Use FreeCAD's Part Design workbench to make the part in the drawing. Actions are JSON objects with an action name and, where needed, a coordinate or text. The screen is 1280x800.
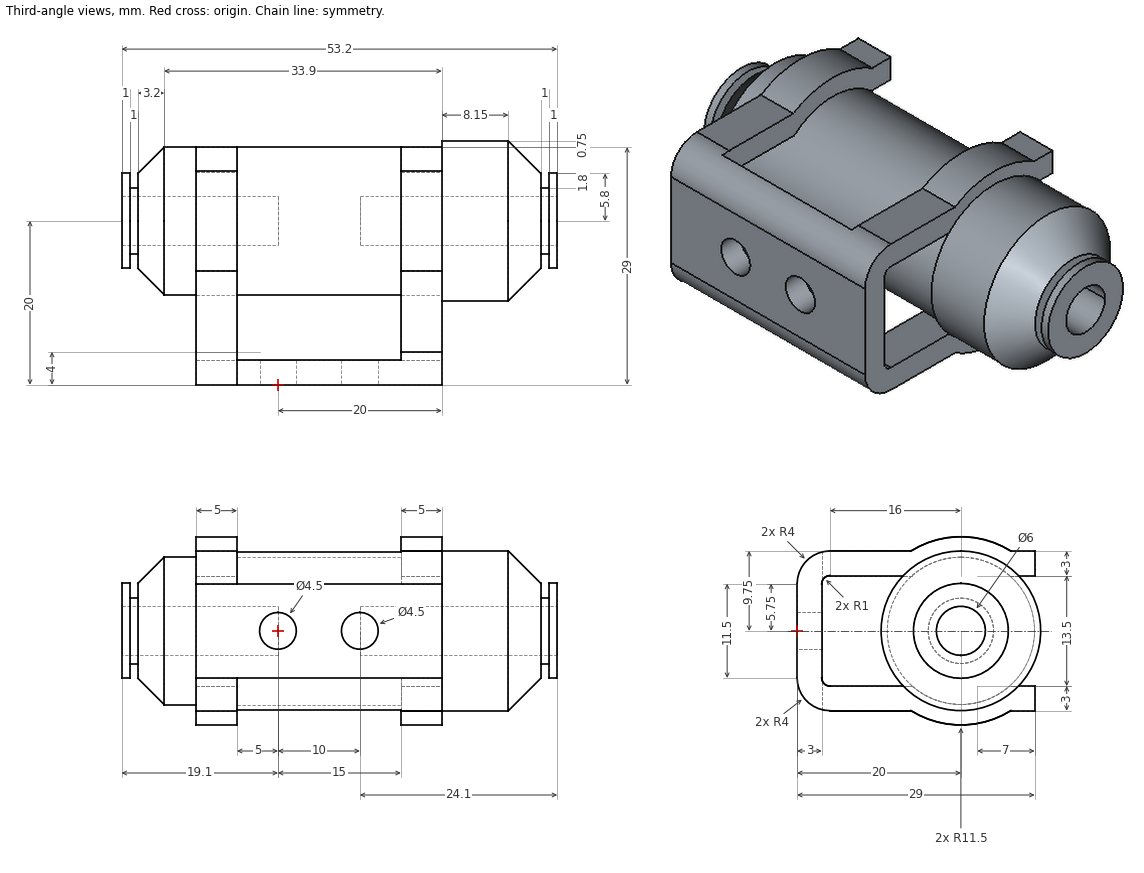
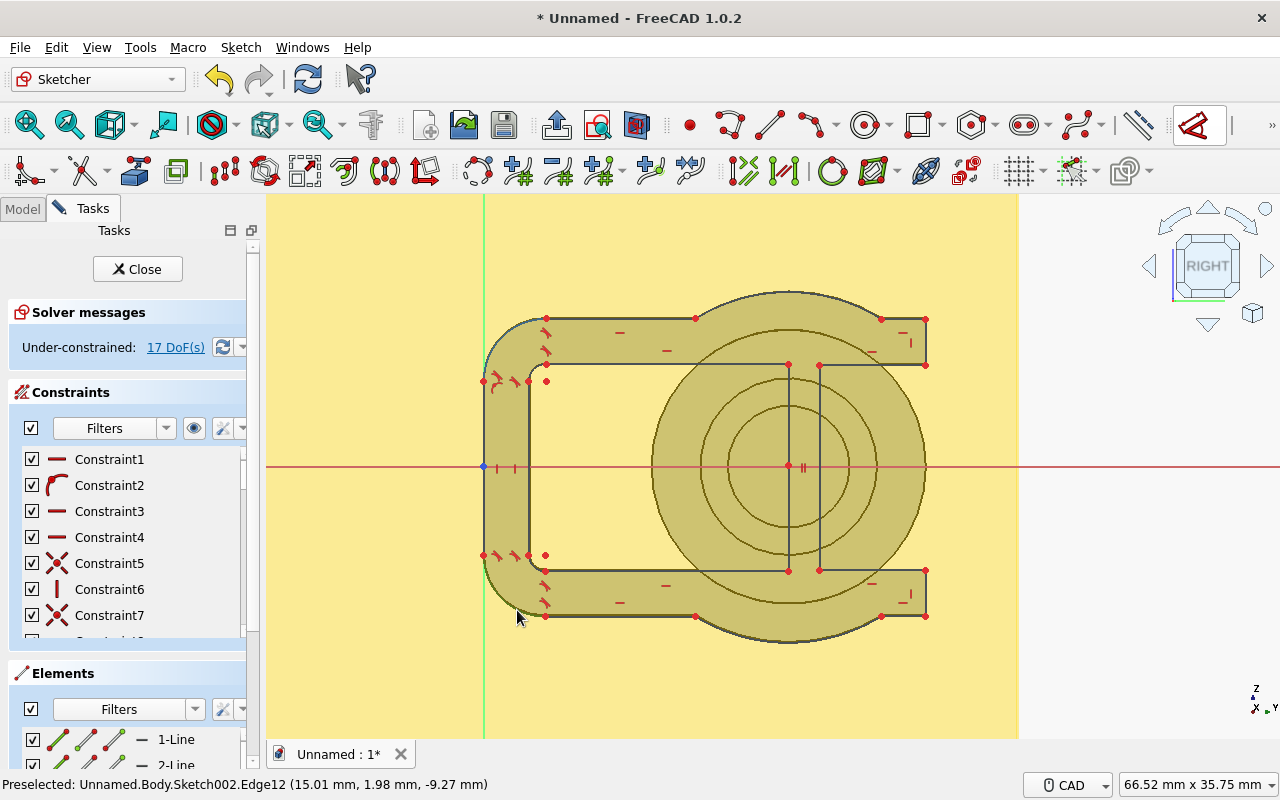
{"action": "key", "text": "e"}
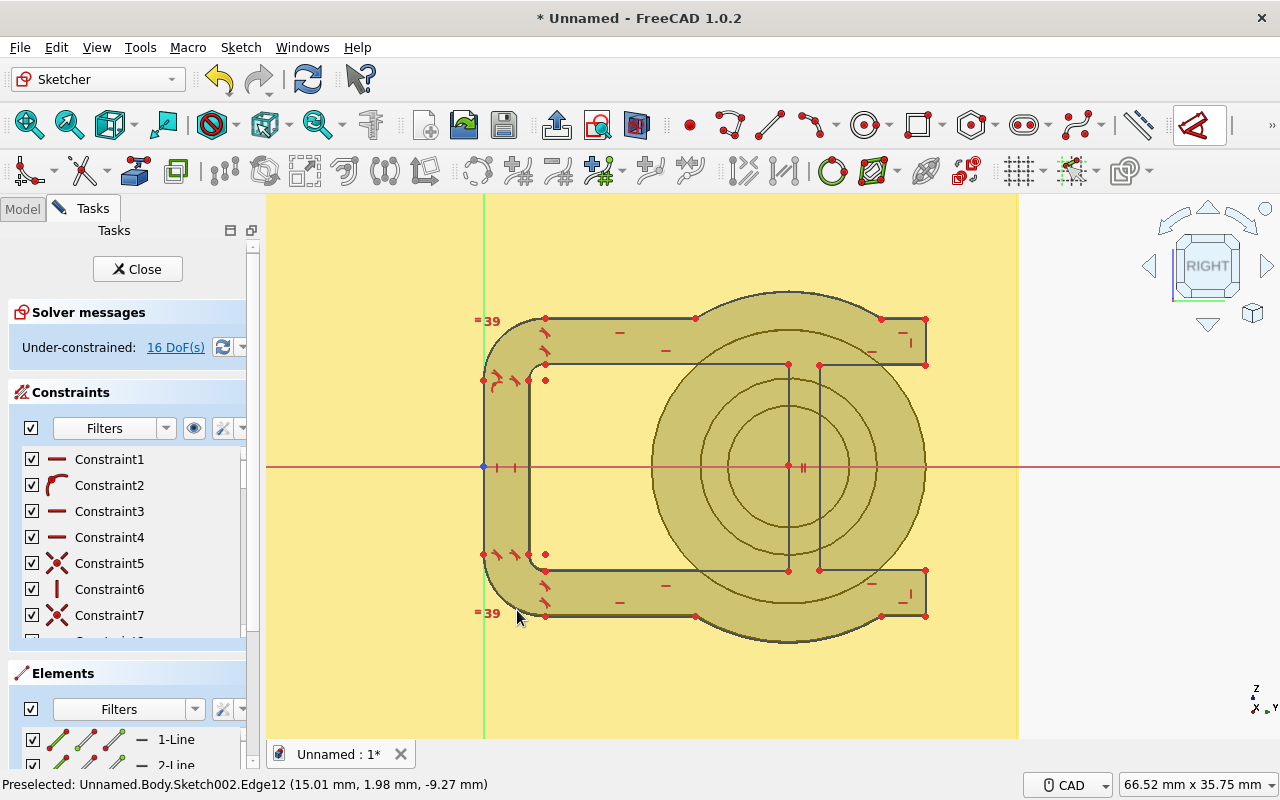
{"action": "left_click", "coordinate": [750, 639]}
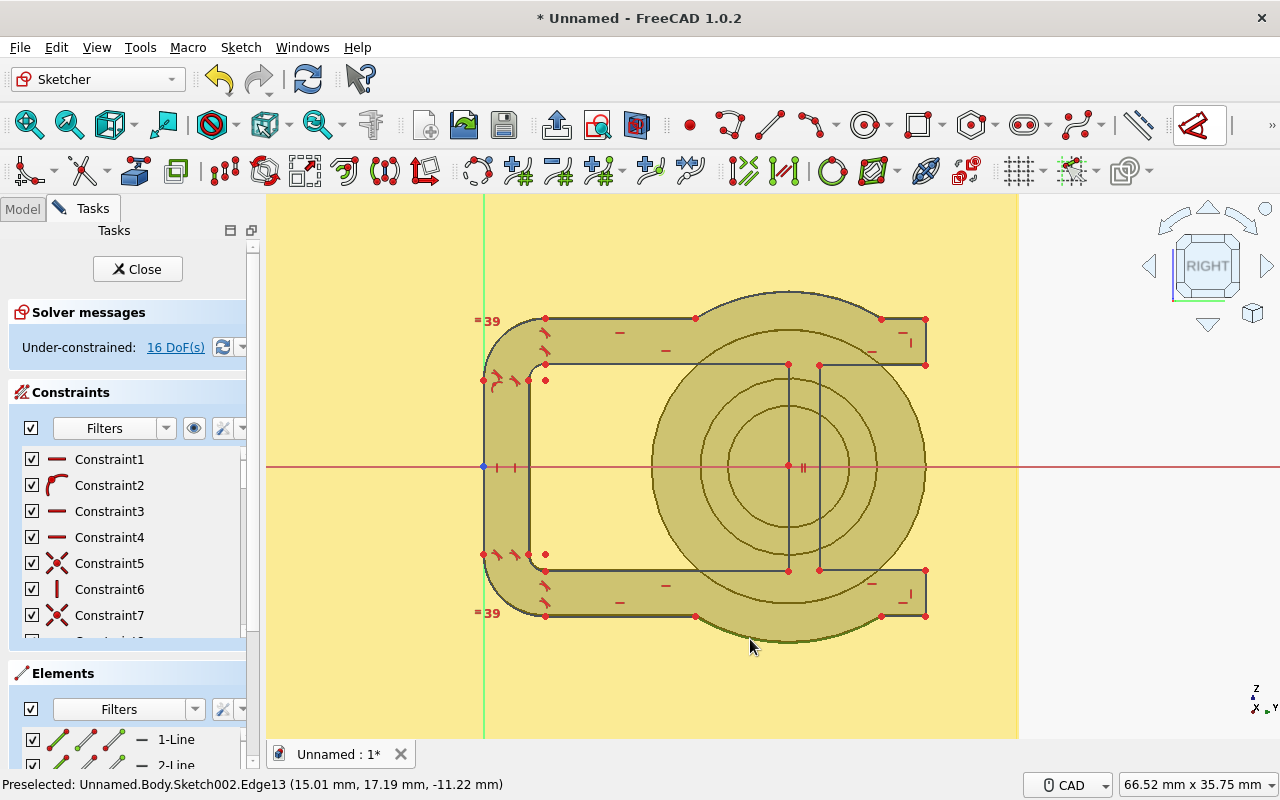
{"action": "left_click", "coordinate": [827, 297]}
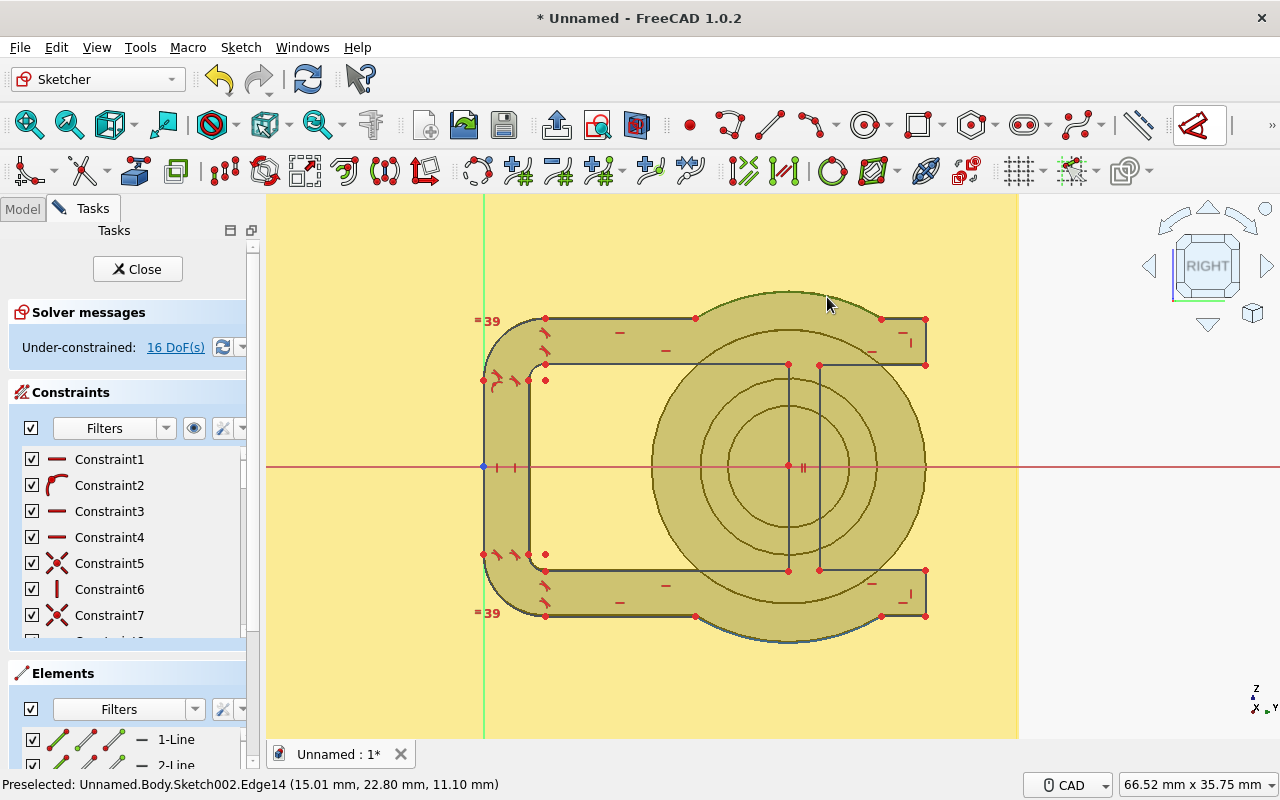
{"action": "key", "text": "e"}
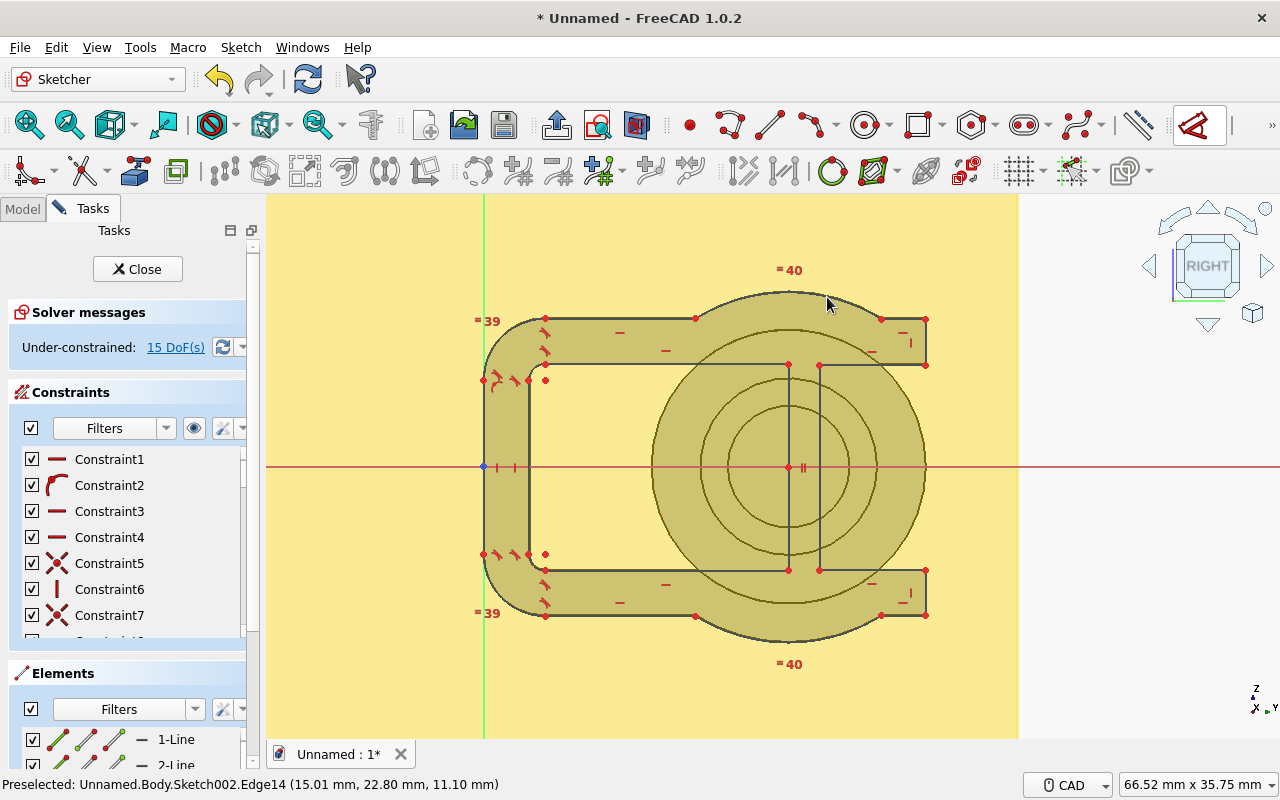
{"action": "left_click", "coordinate": [788, 467]}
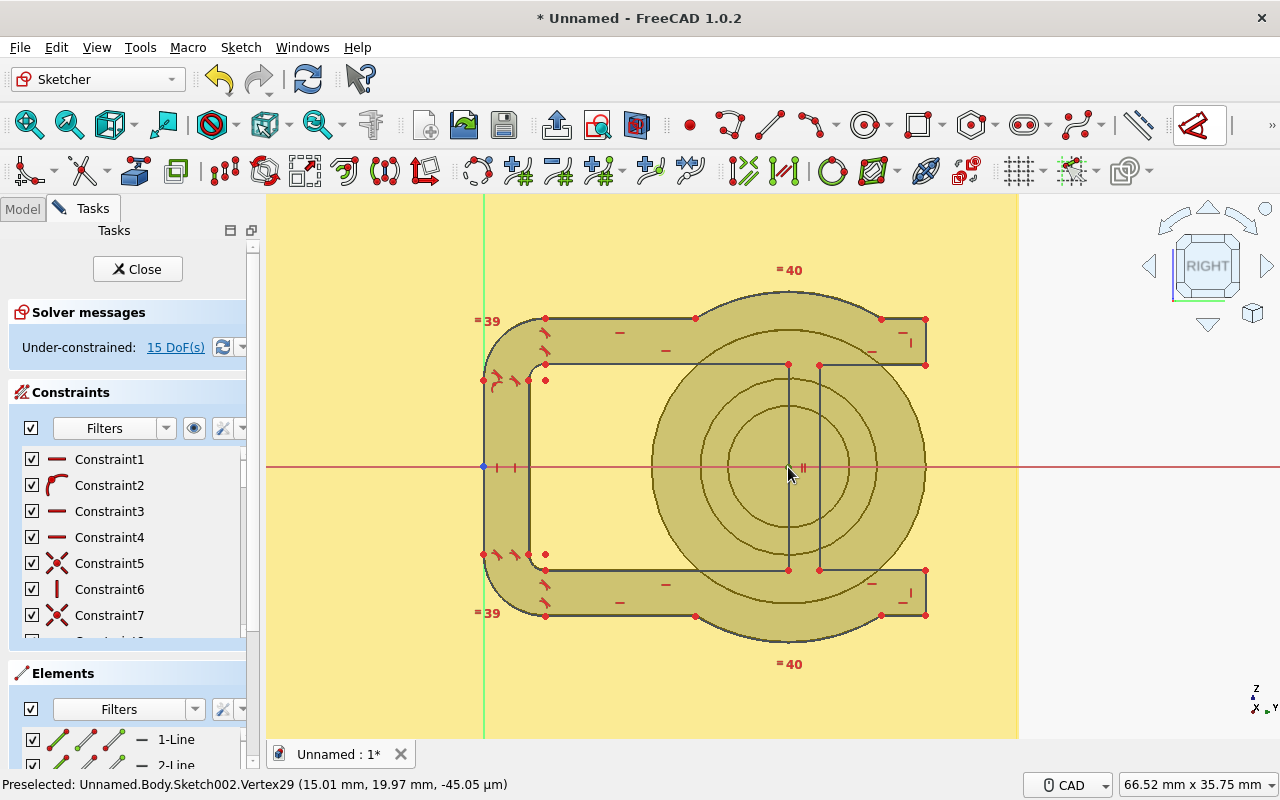
{"action": "left_click", "coordinate": [353, 467]}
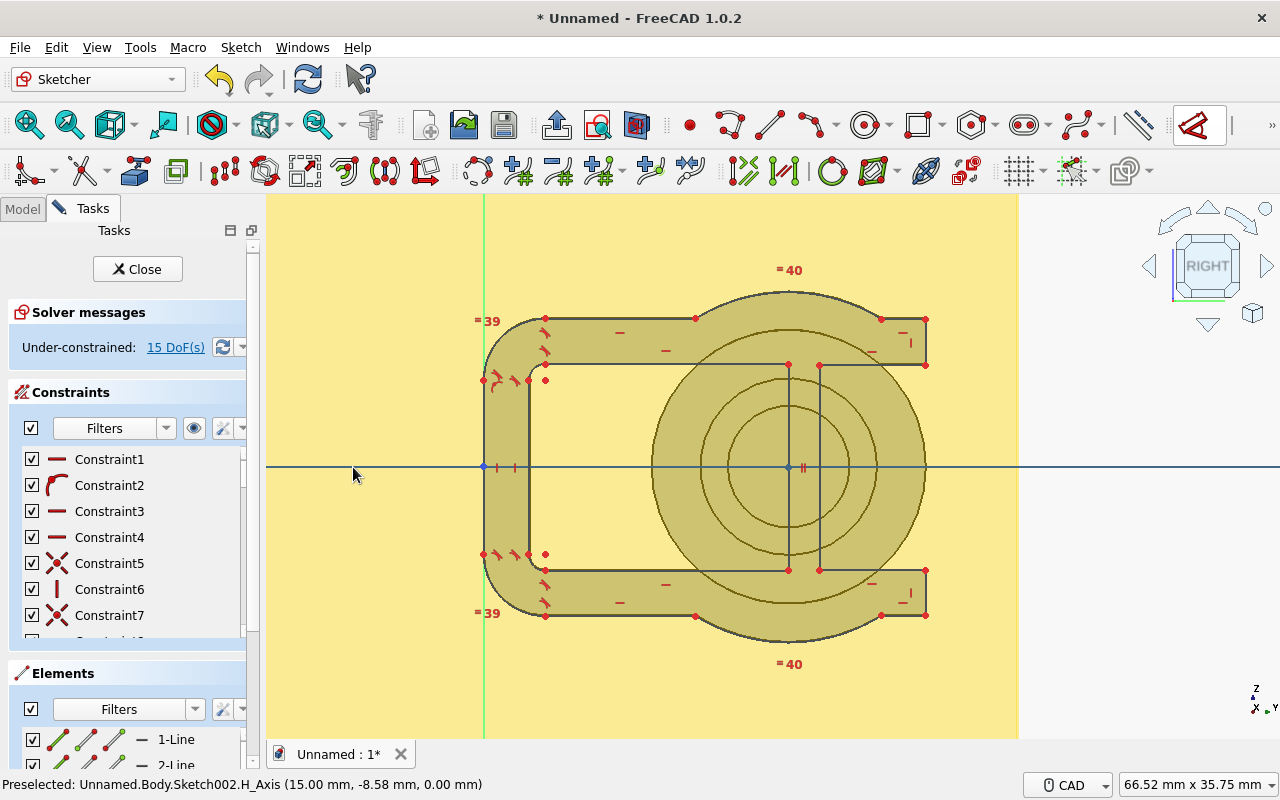
{"action": "key", "text": "c"}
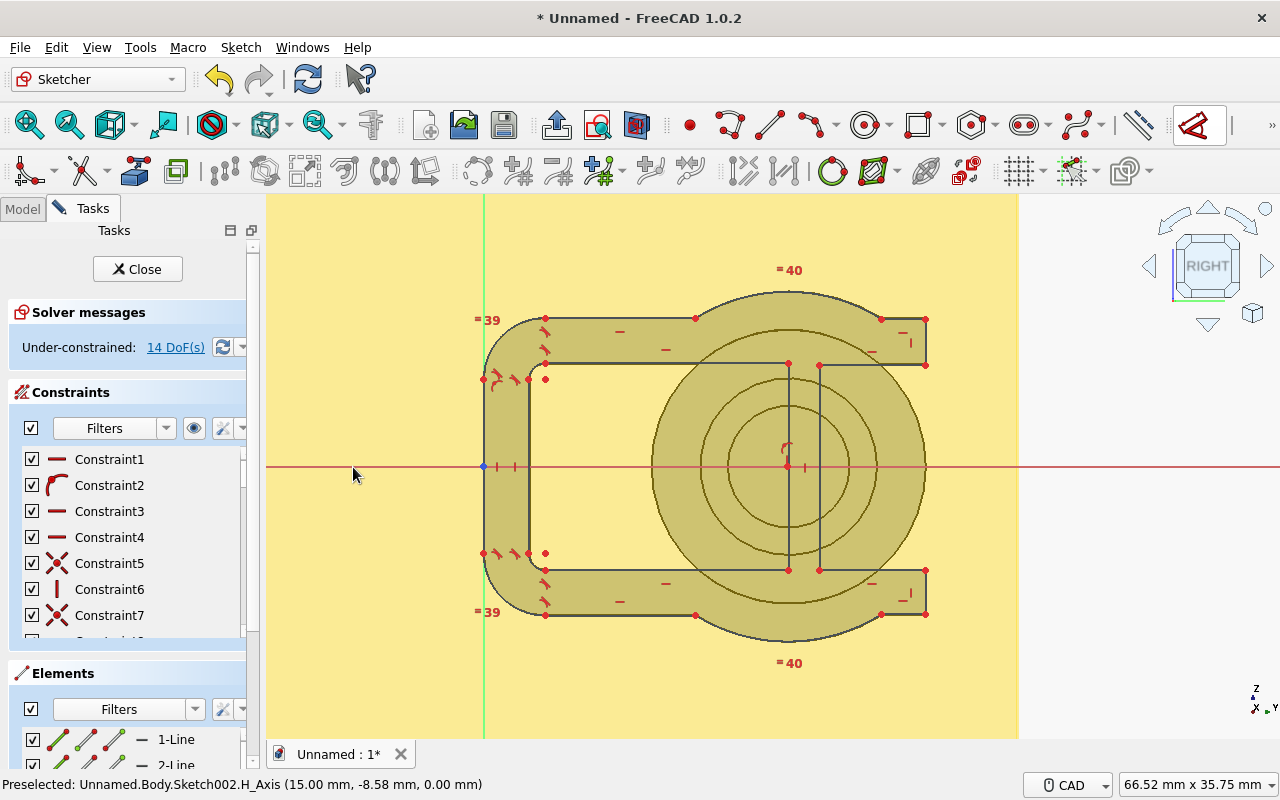
{"action": "left_click", "coordinate": [926, 570]}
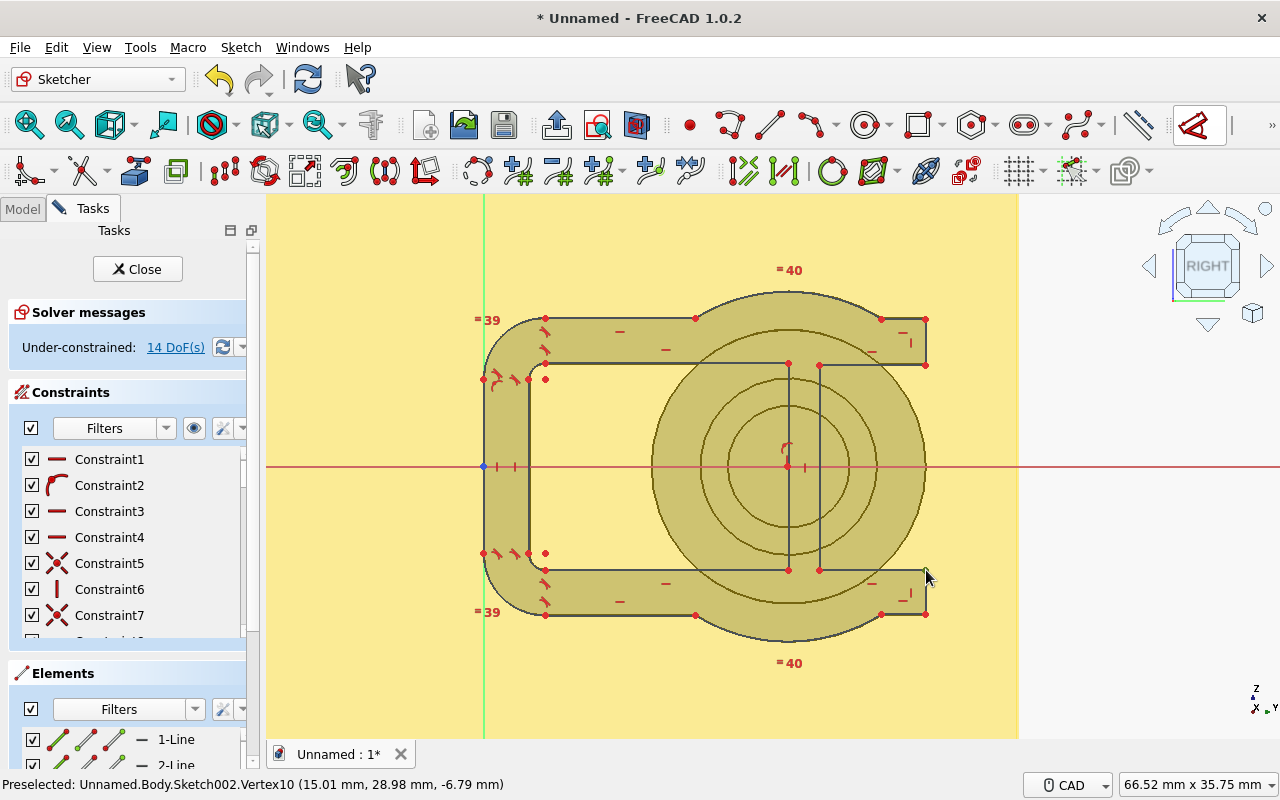
{"action": "left_click", "coordinate": [926, 365]}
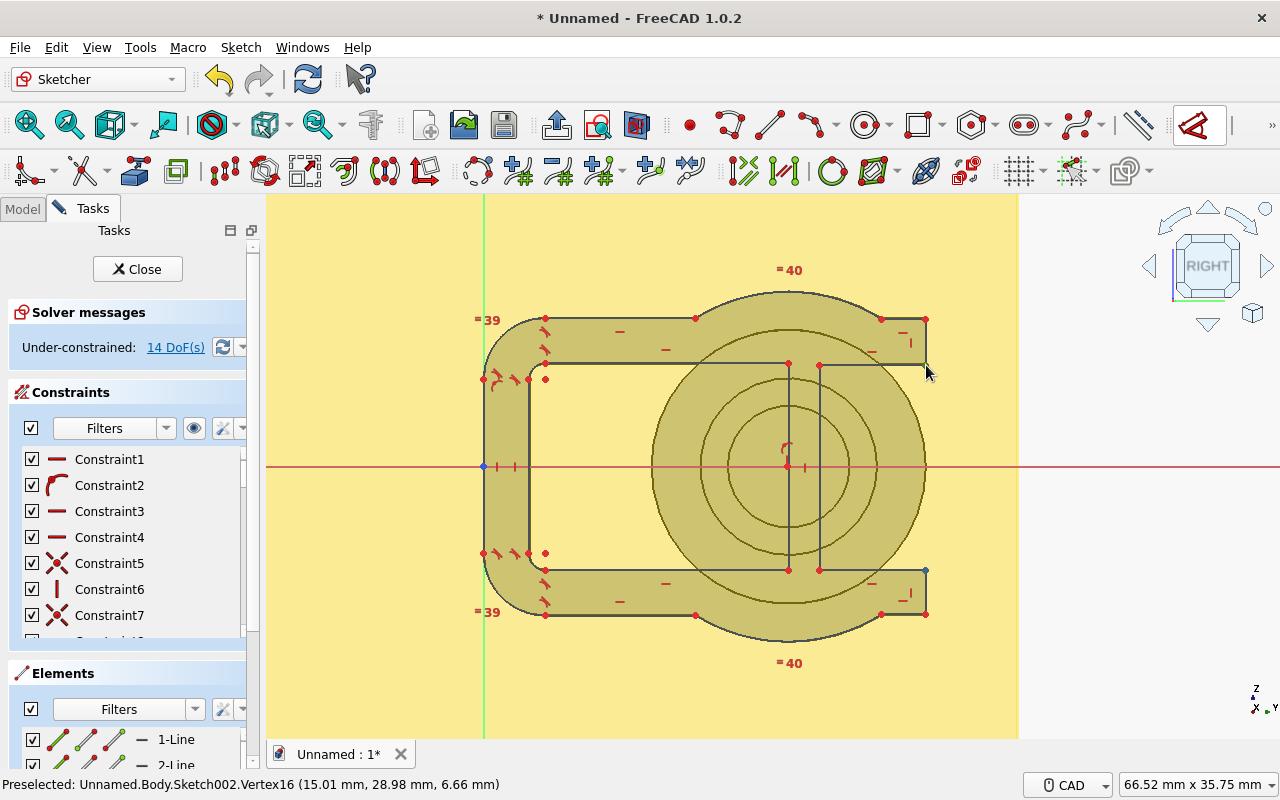
{"action": "left_click", "coordinate": [353, 467]}